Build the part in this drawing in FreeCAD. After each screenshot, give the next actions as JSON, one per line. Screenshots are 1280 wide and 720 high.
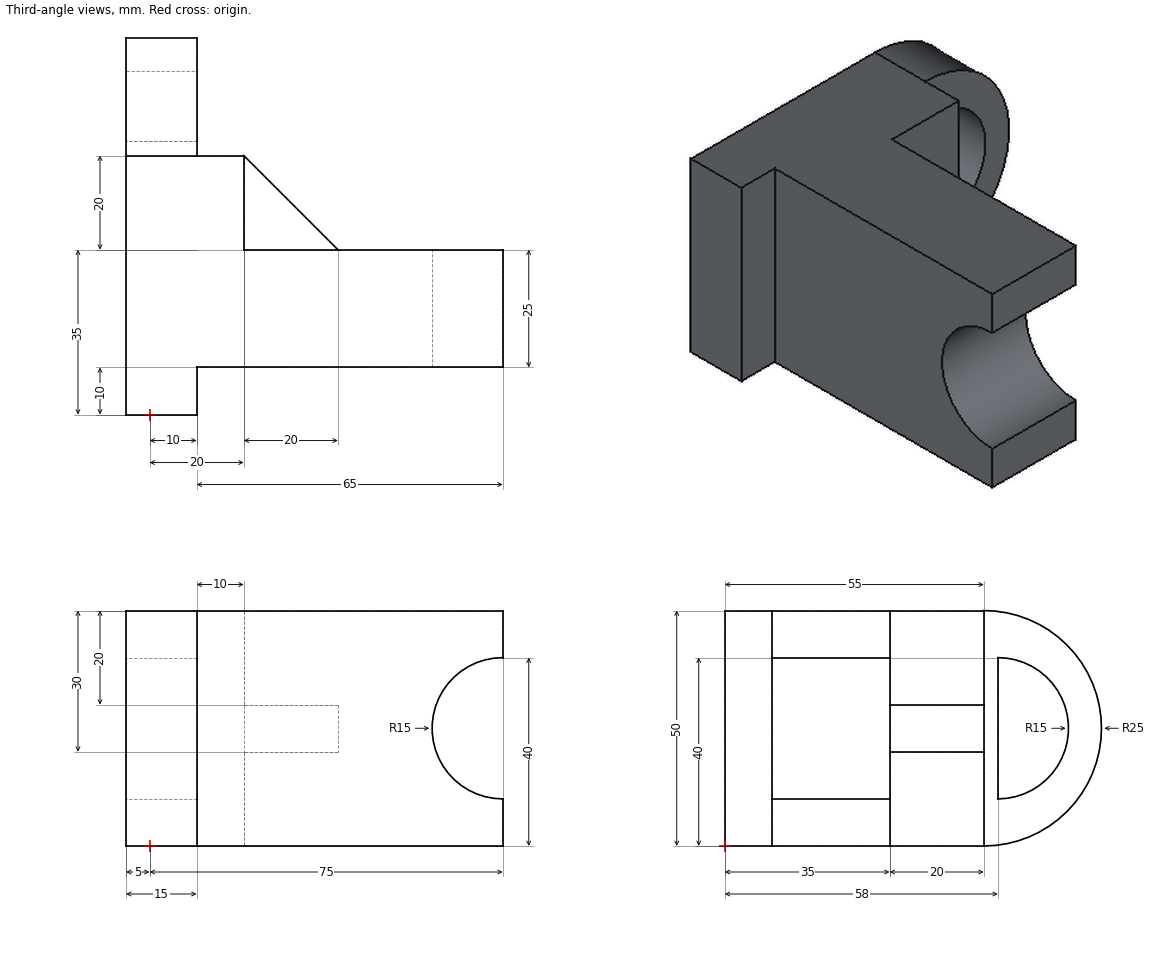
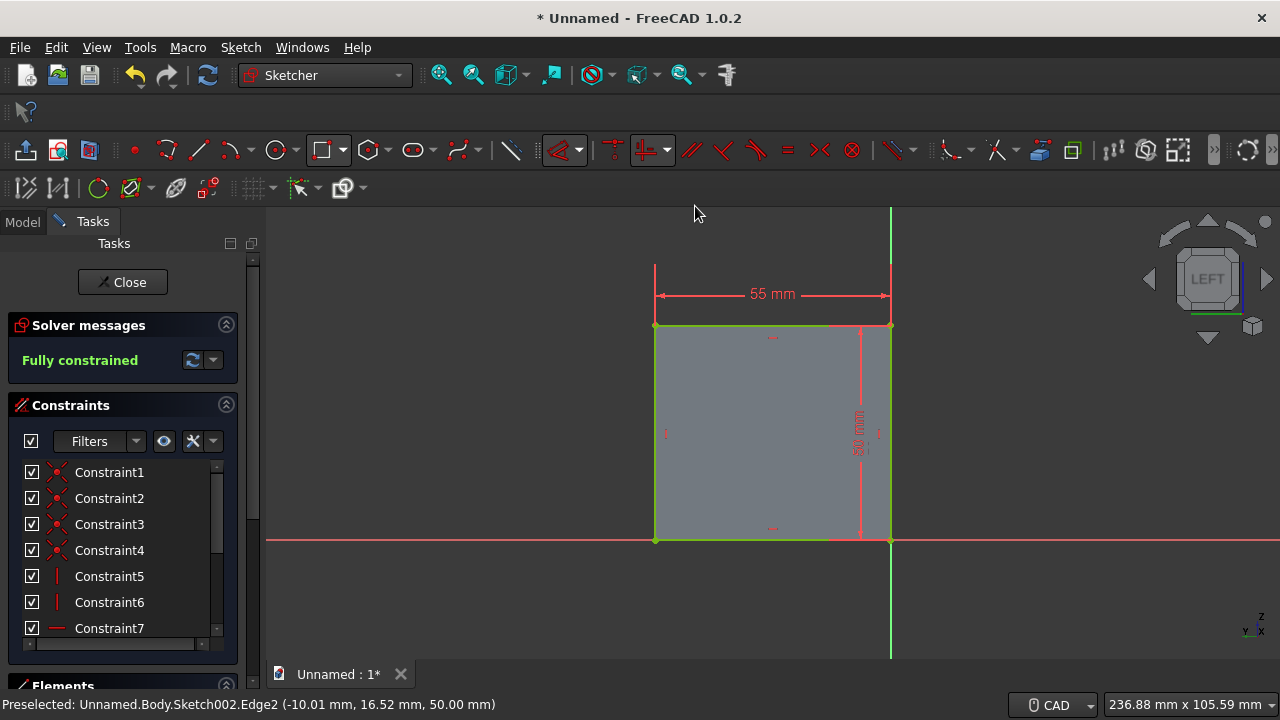
{"action": "left_click", "coordinate": [123, 282]}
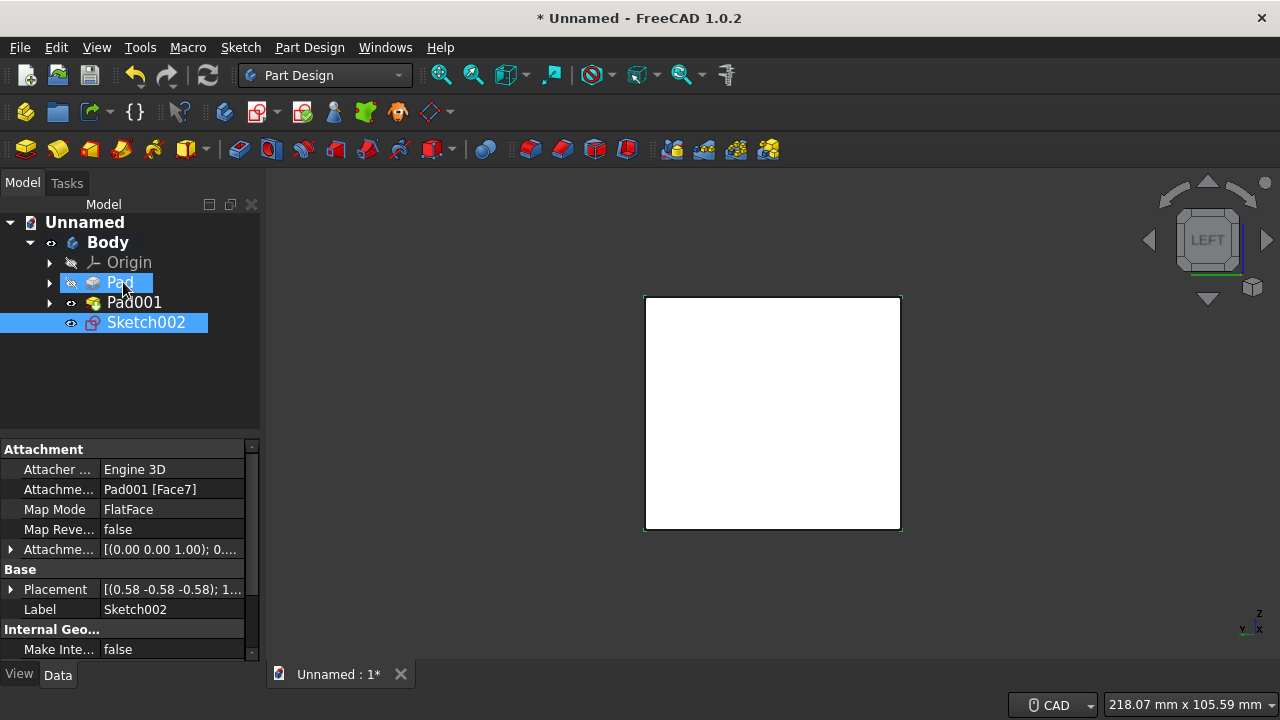
{"action": "left_click", "coordinate": [240, 150]}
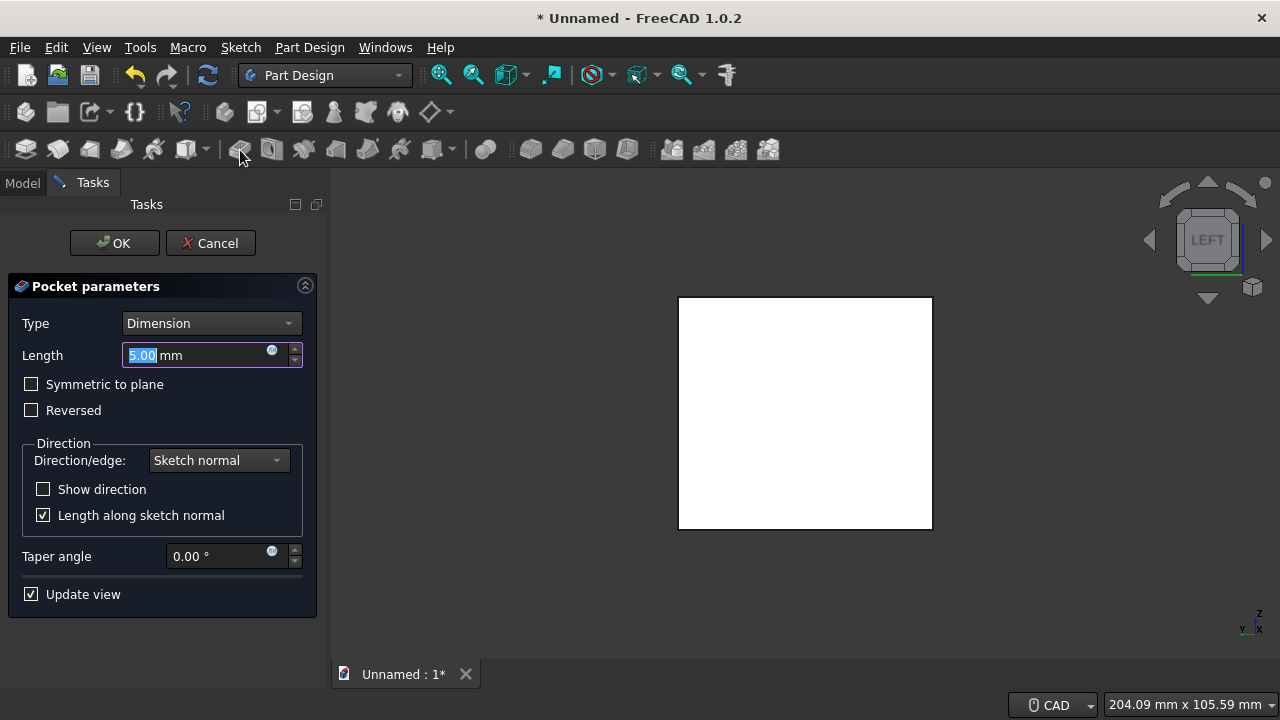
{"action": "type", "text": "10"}
{"action": "key", "text": "Tab"}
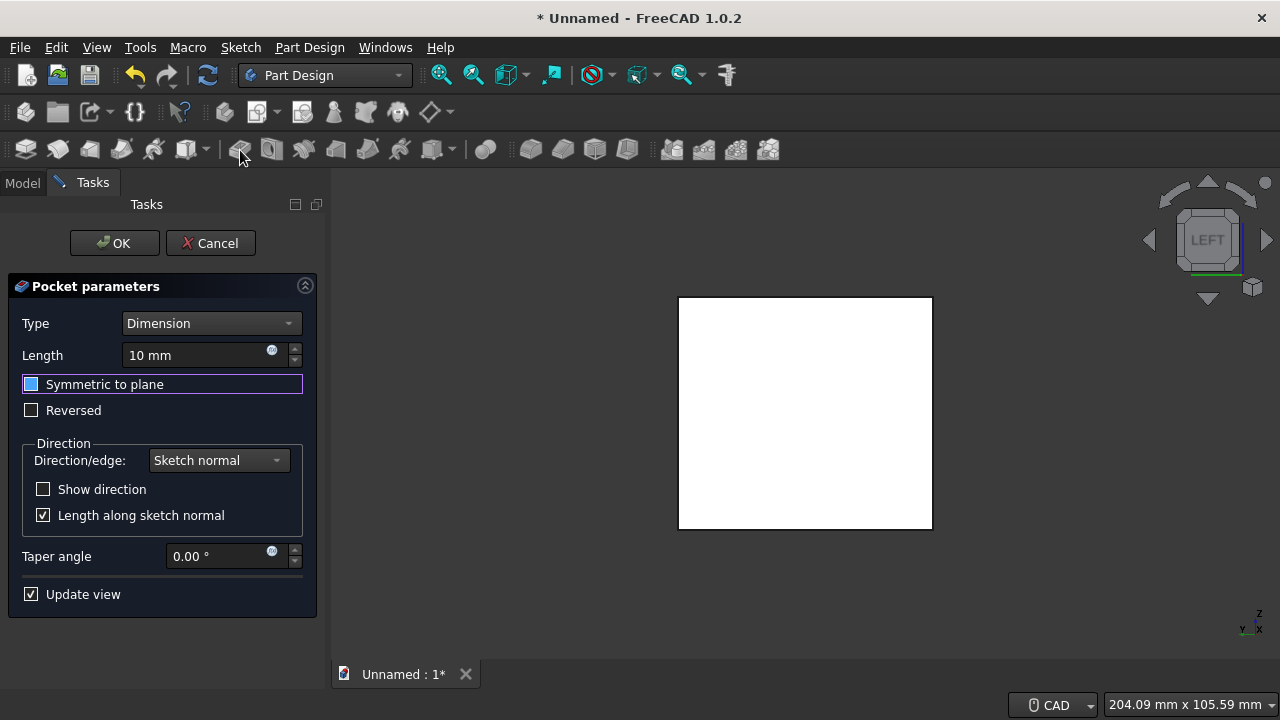
{"action": "left_click", "coordinate": [115, 243]}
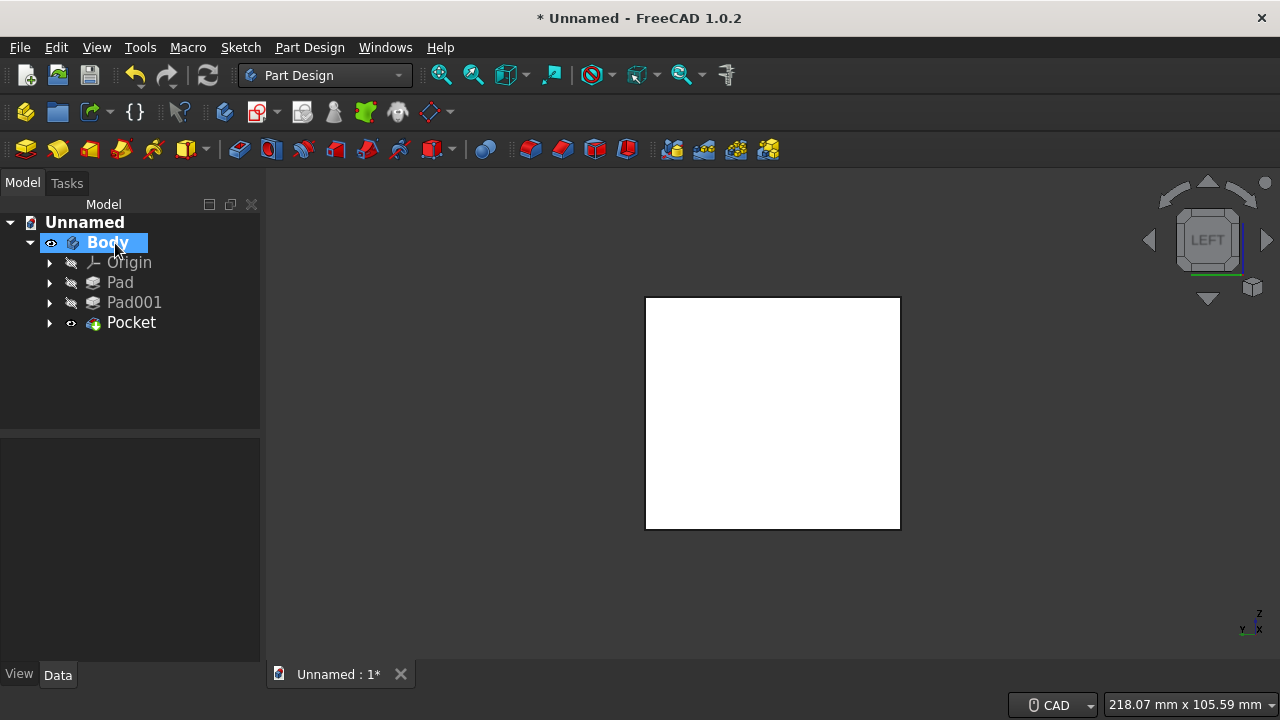
{"action": "left_click", "coordinate": [773, 413]}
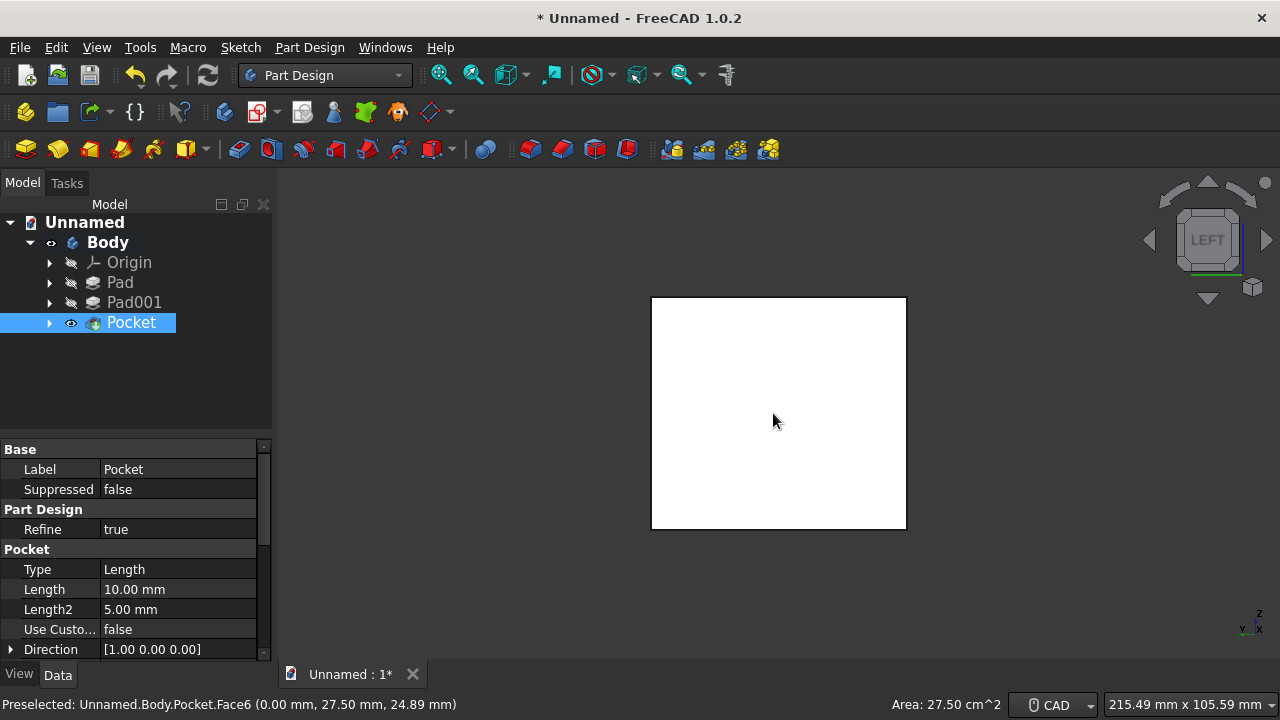
{"action": "left_click", "coordinate": [258, 112]}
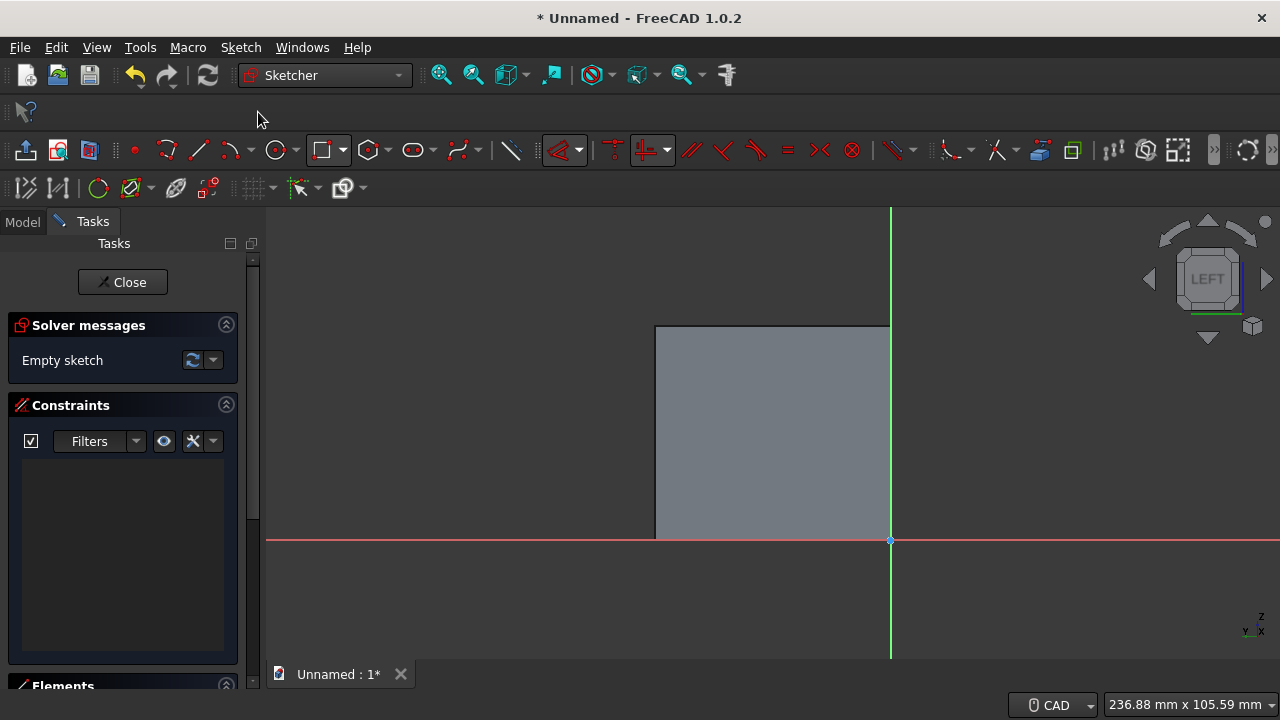
{"action": "key", "text": "g r"}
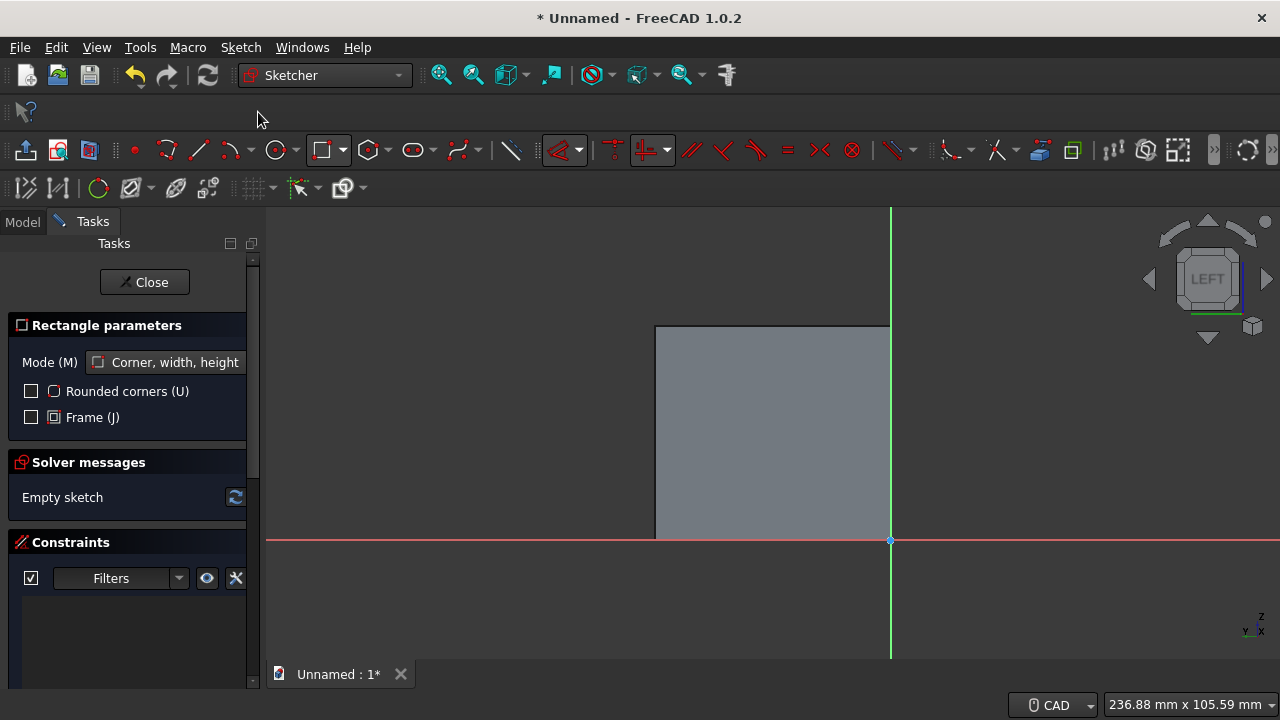
{"action": "left_click", "coordinate": [891, 540]}
{"action": "left_click", "coordinate": [655, 326]}
{"action": "key", "text": "Escape"}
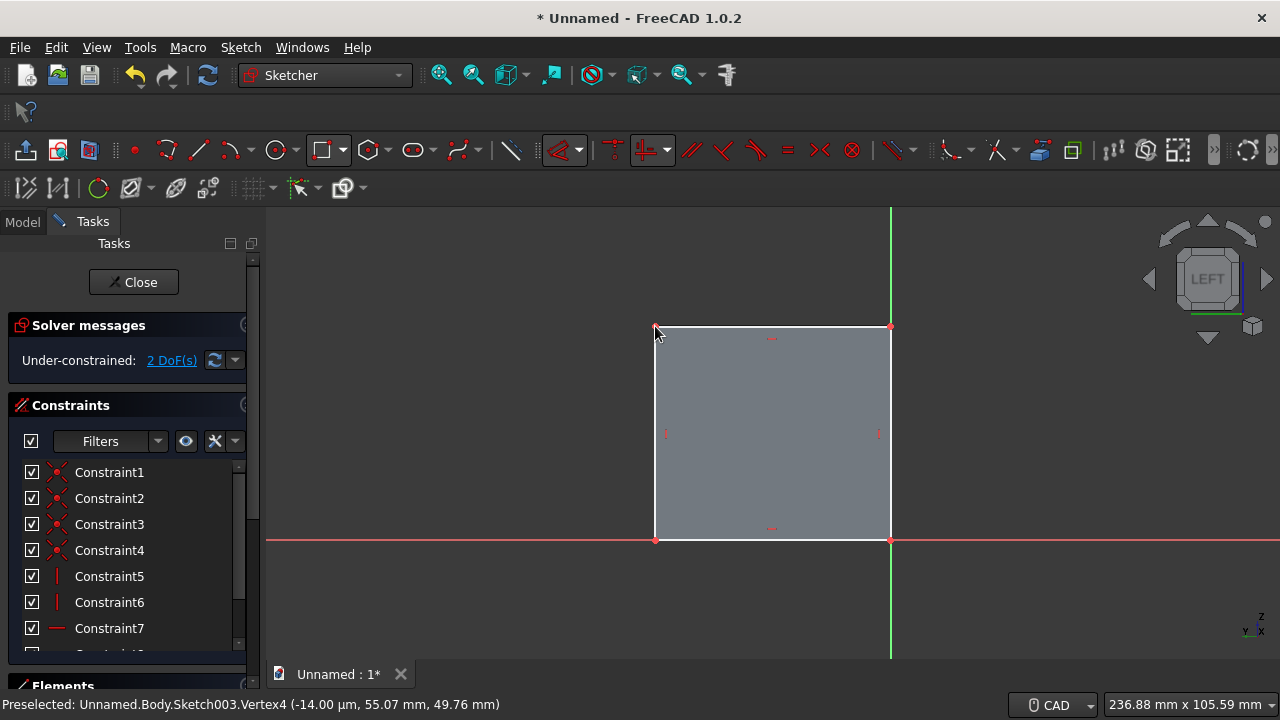
{"action": "left_click", "coordinate": [891, 476]}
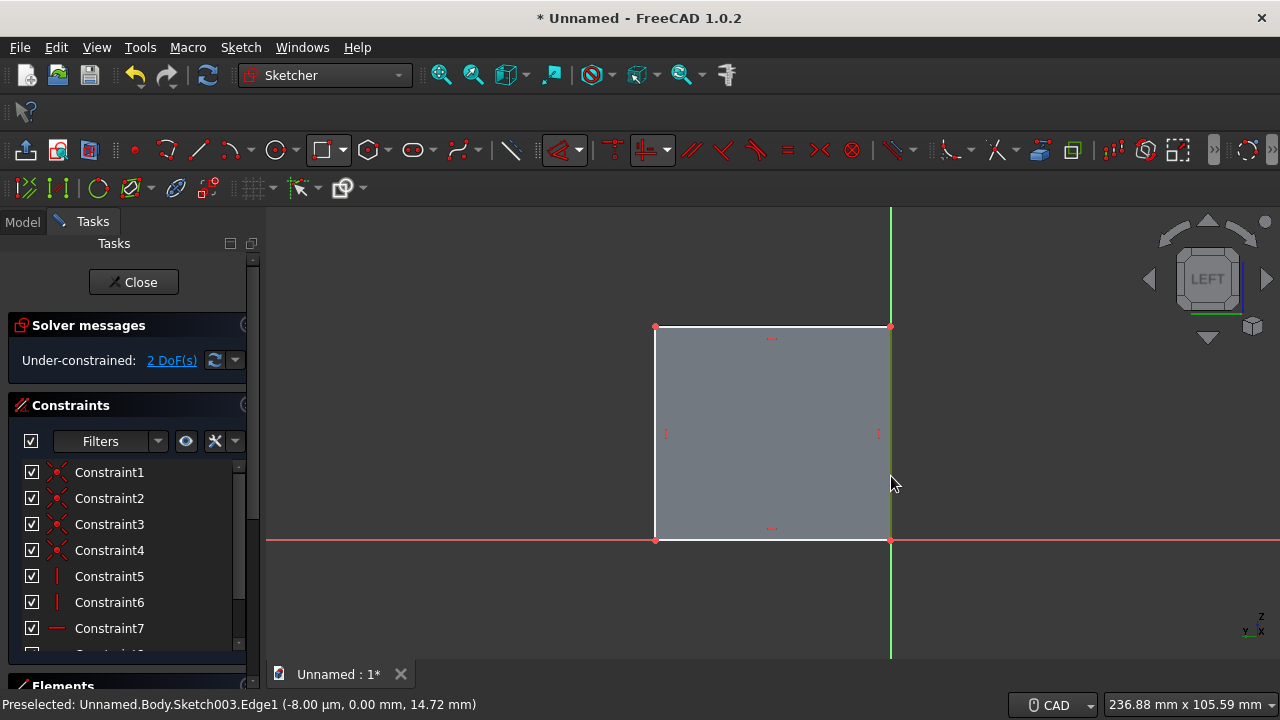
{"action": "key", "text": "i"}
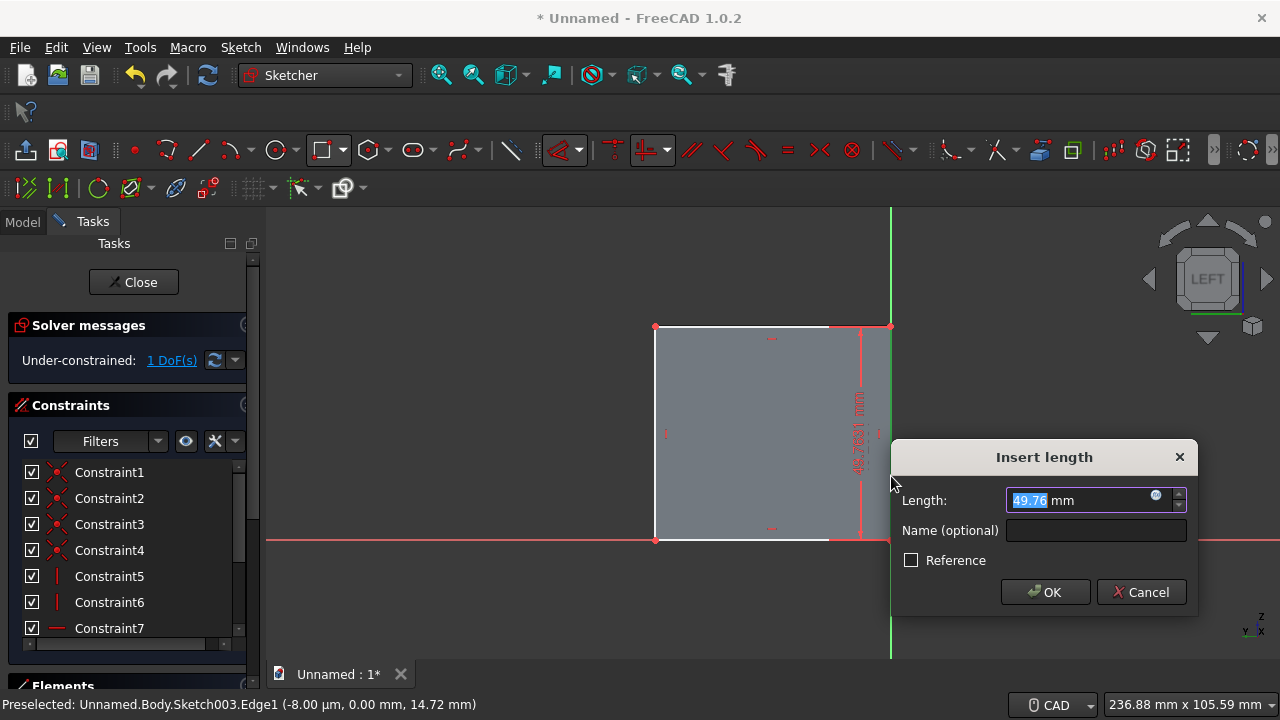
{"action": "type", "text": "50"}
{"action": "key", "text": "Return"}